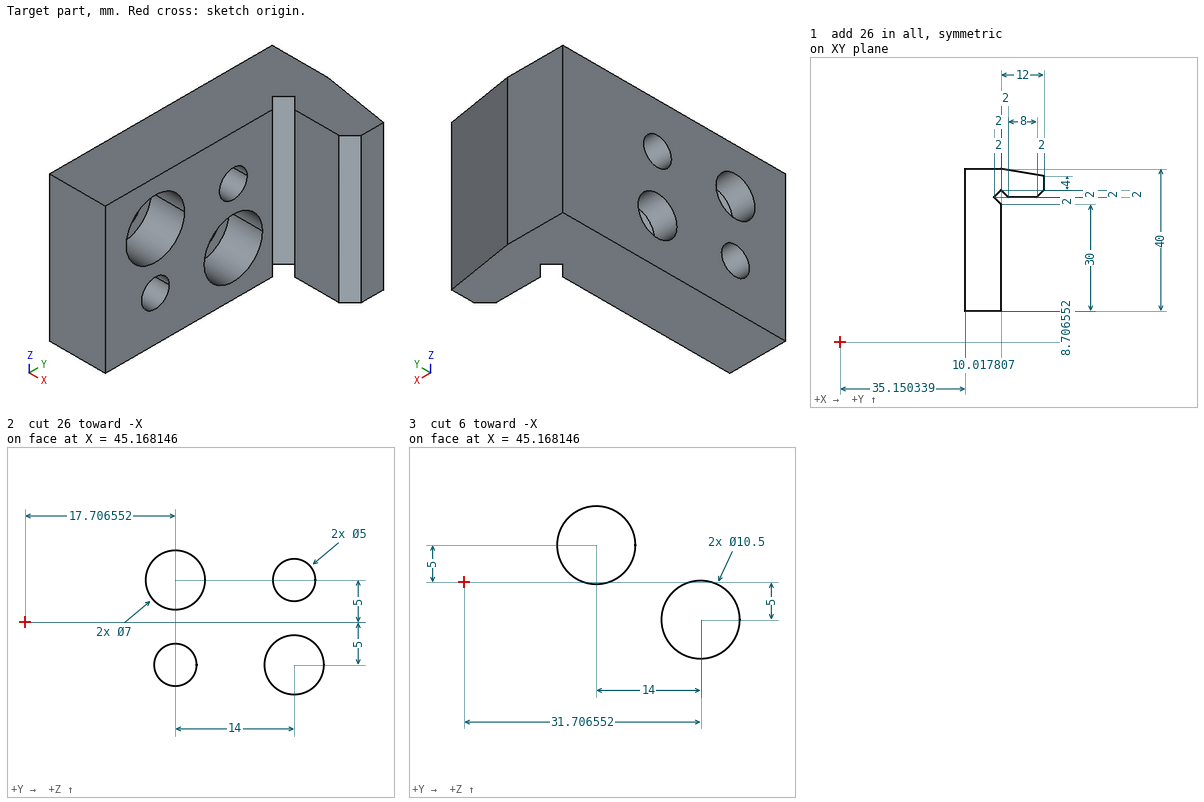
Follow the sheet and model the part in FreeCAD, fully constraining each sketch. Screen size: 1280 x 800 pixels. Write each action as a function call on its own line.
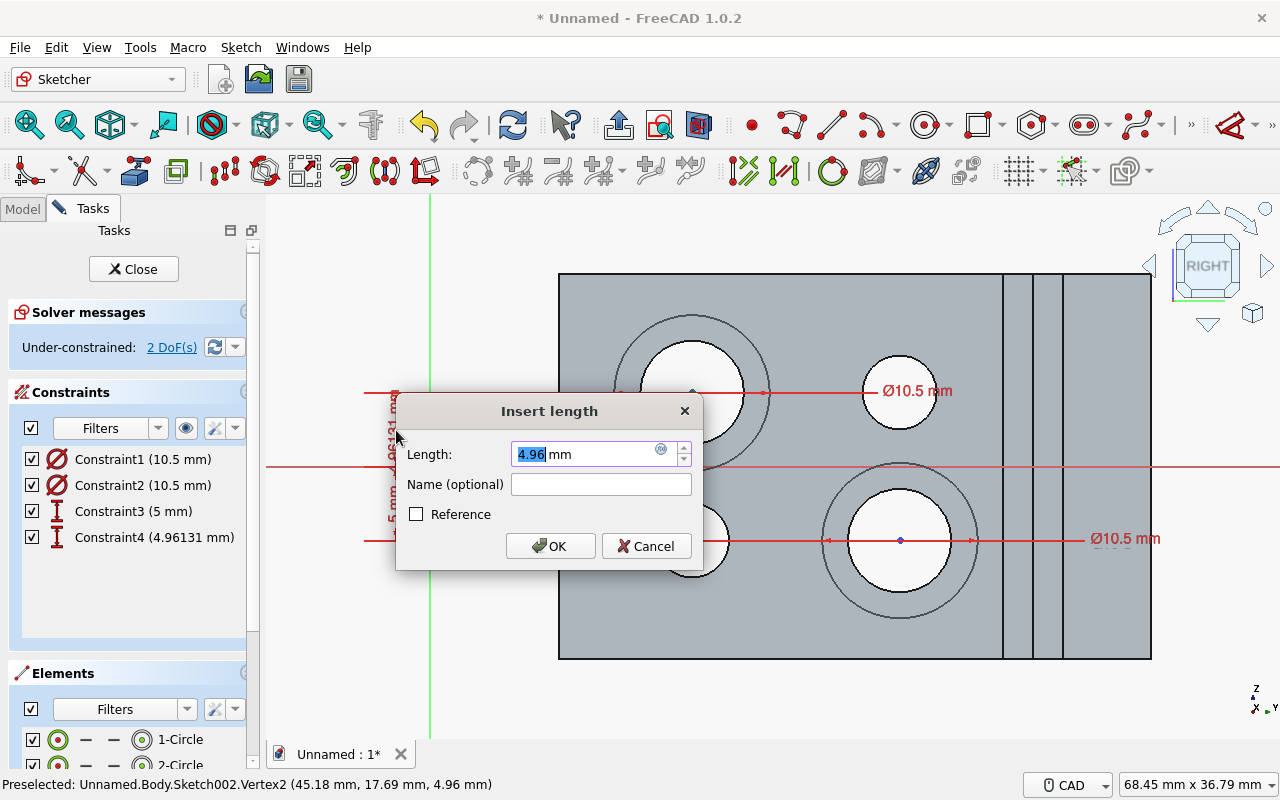
text(5)
key(Return)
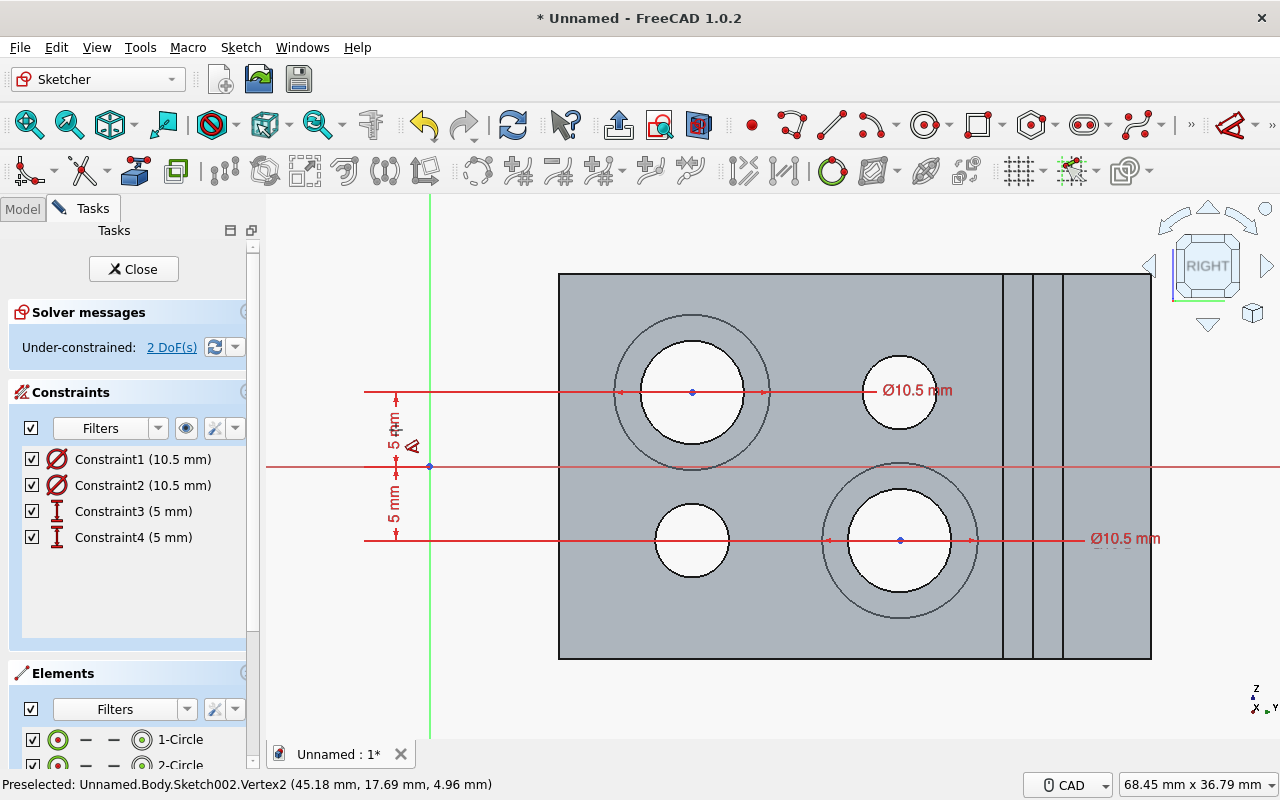
click(900, 541)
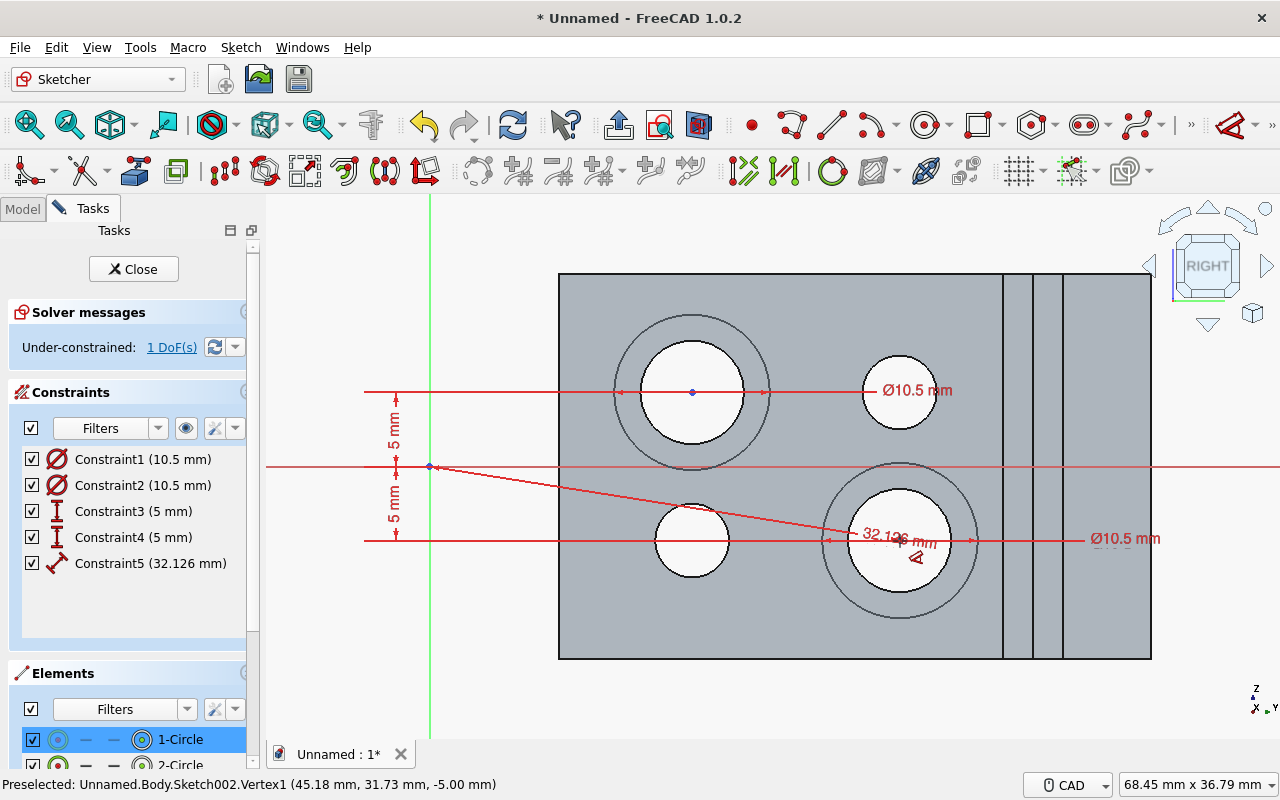
click(692, 392)
click(796, 575)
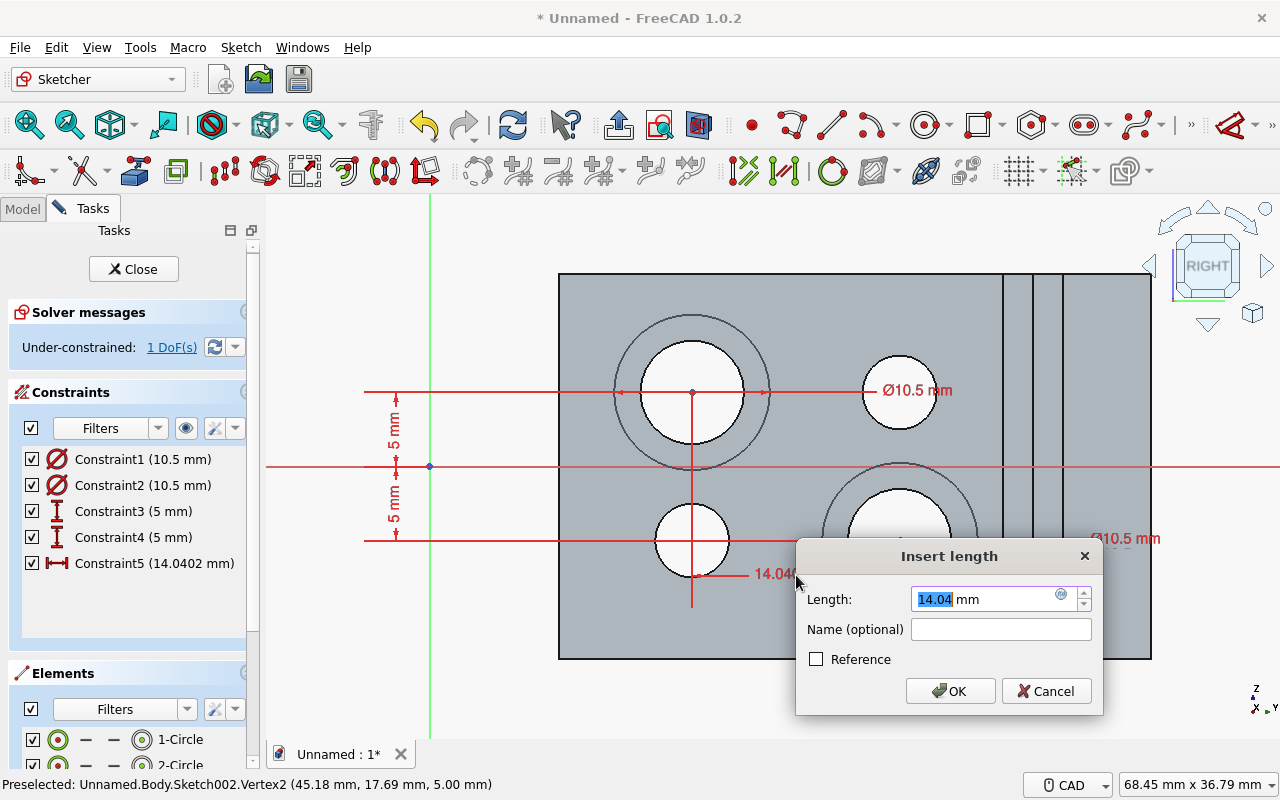
text(14)
key(Return)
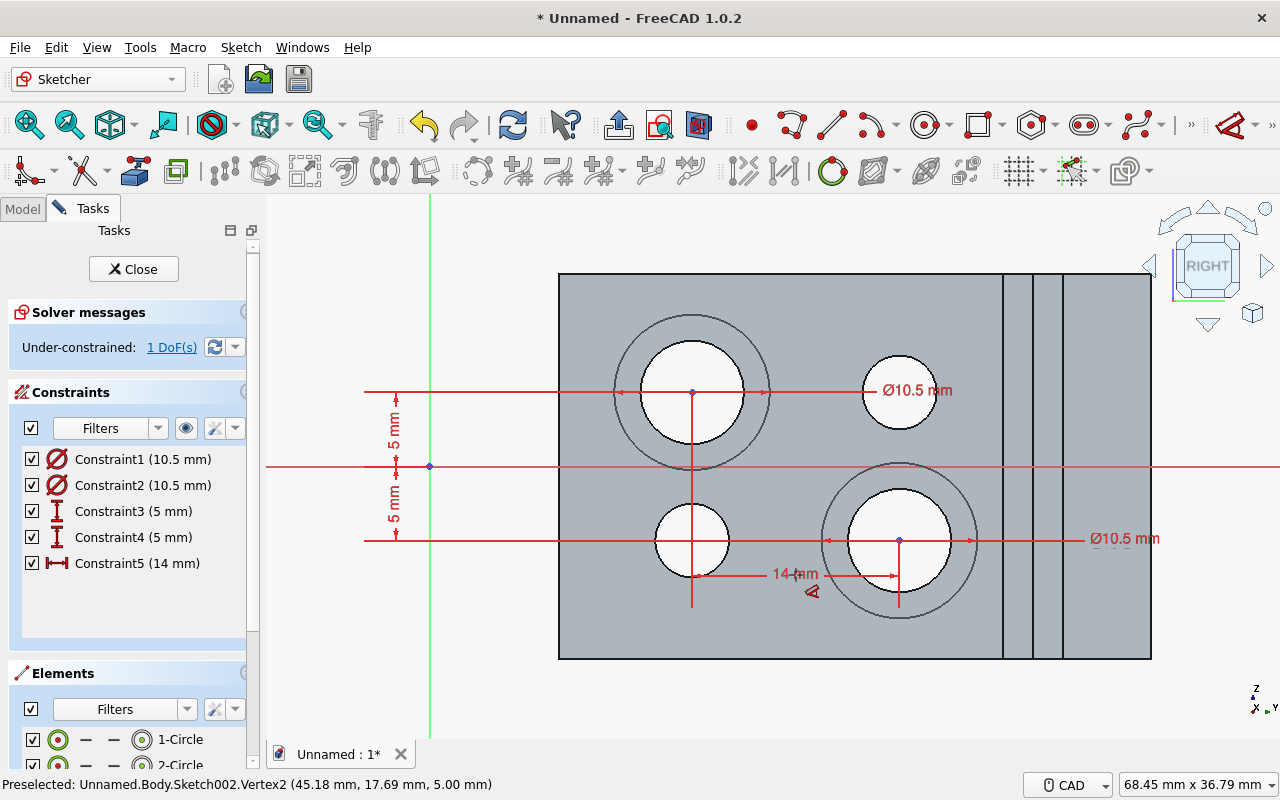
click(899, 541)
click(665, 575)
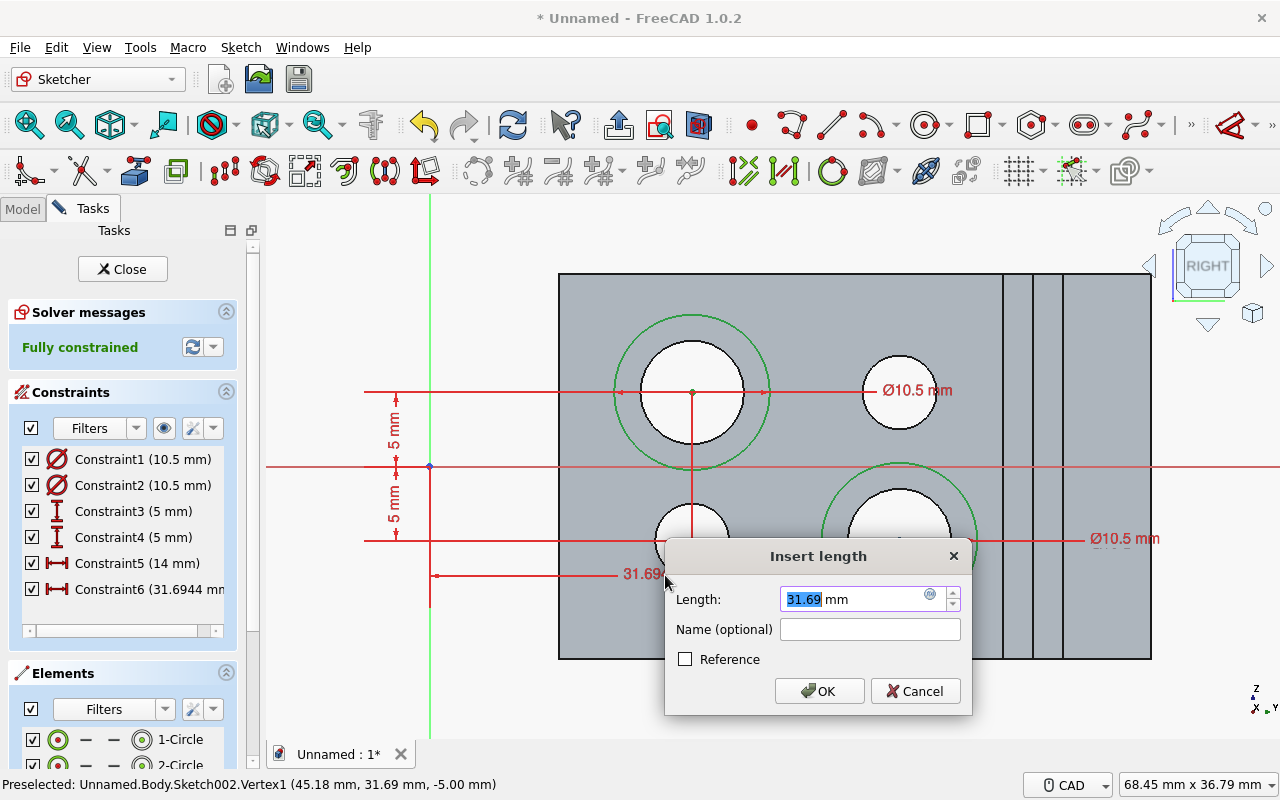
text(31.706552)
key(Return)
key(Escape)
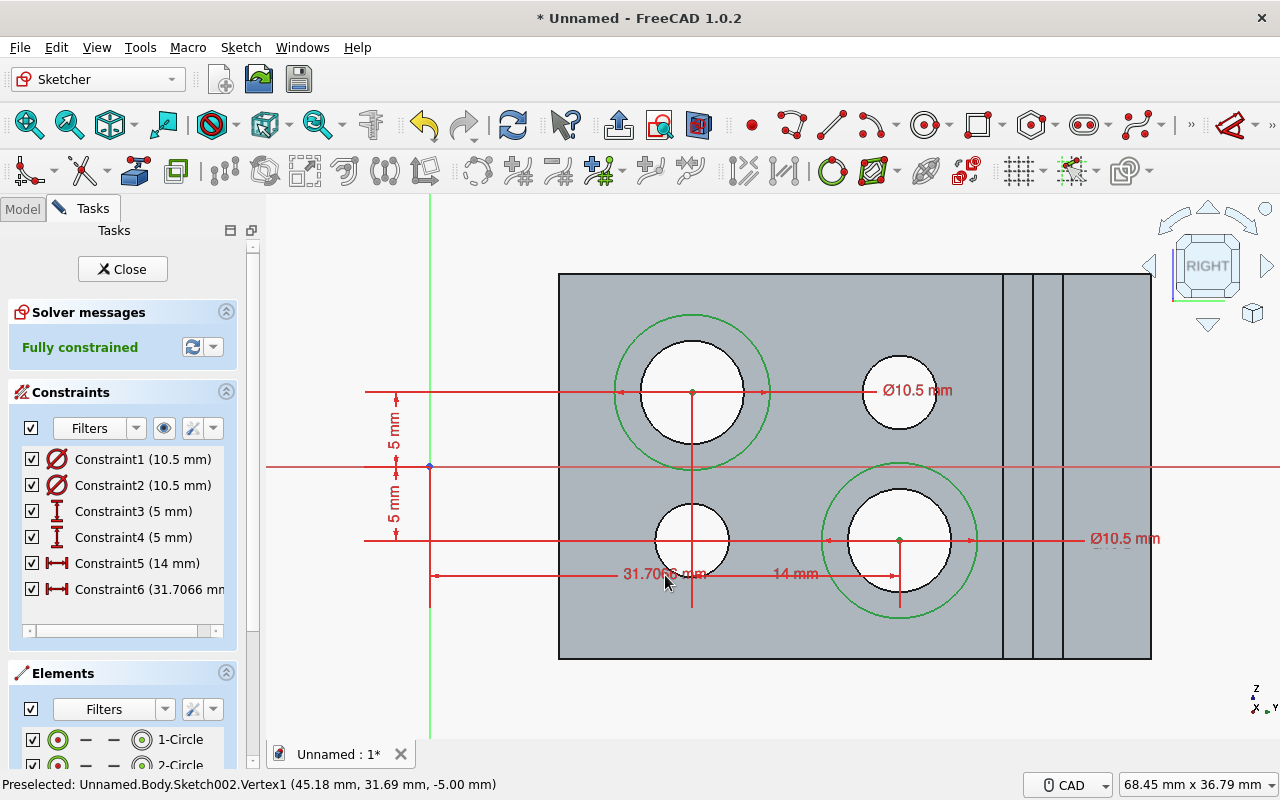
click(123, 269)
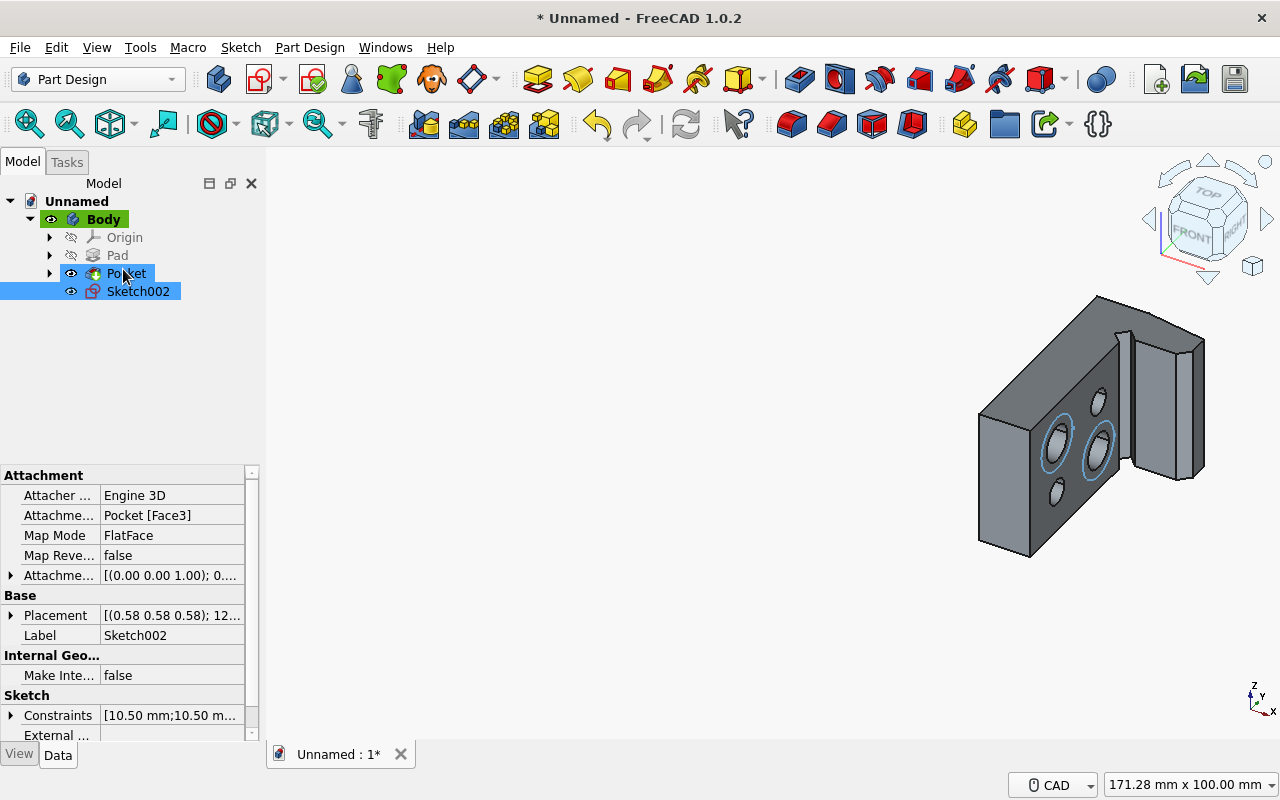
click(800, 80)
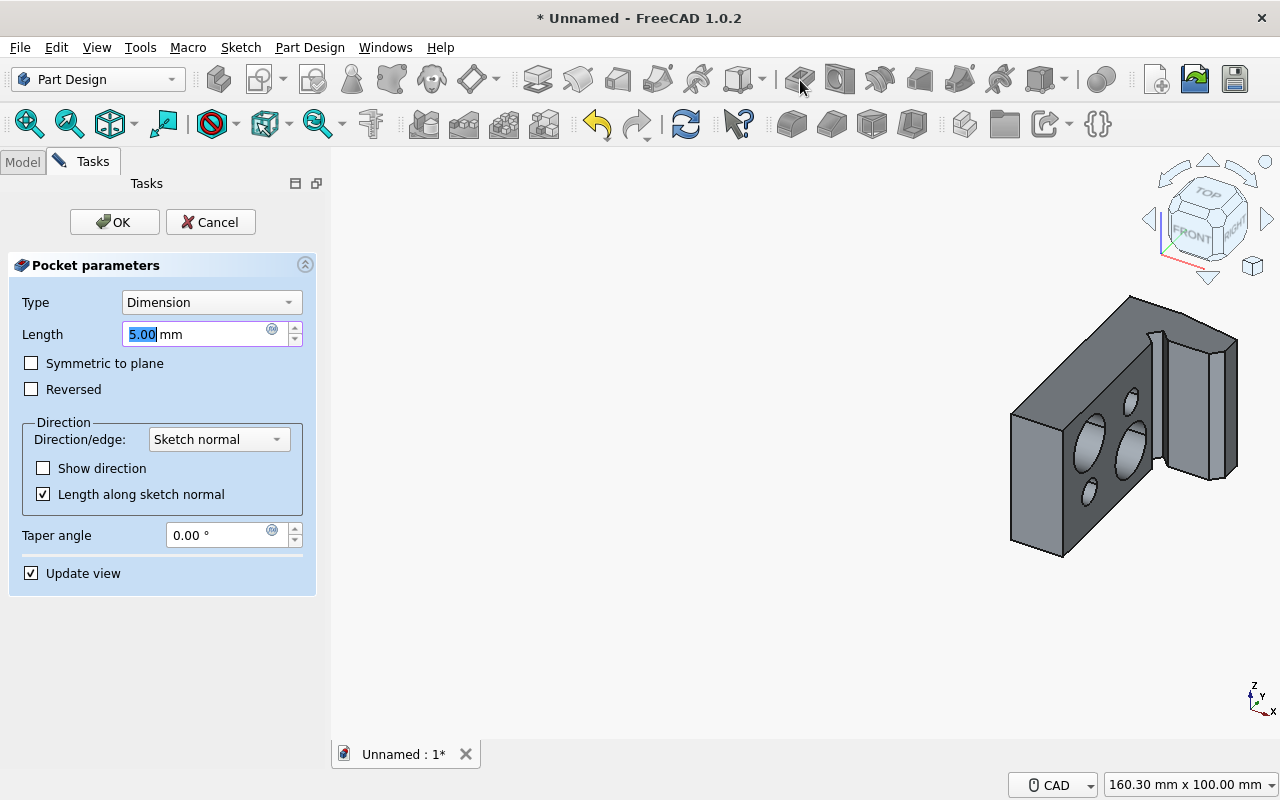
text(6)
key(Tab)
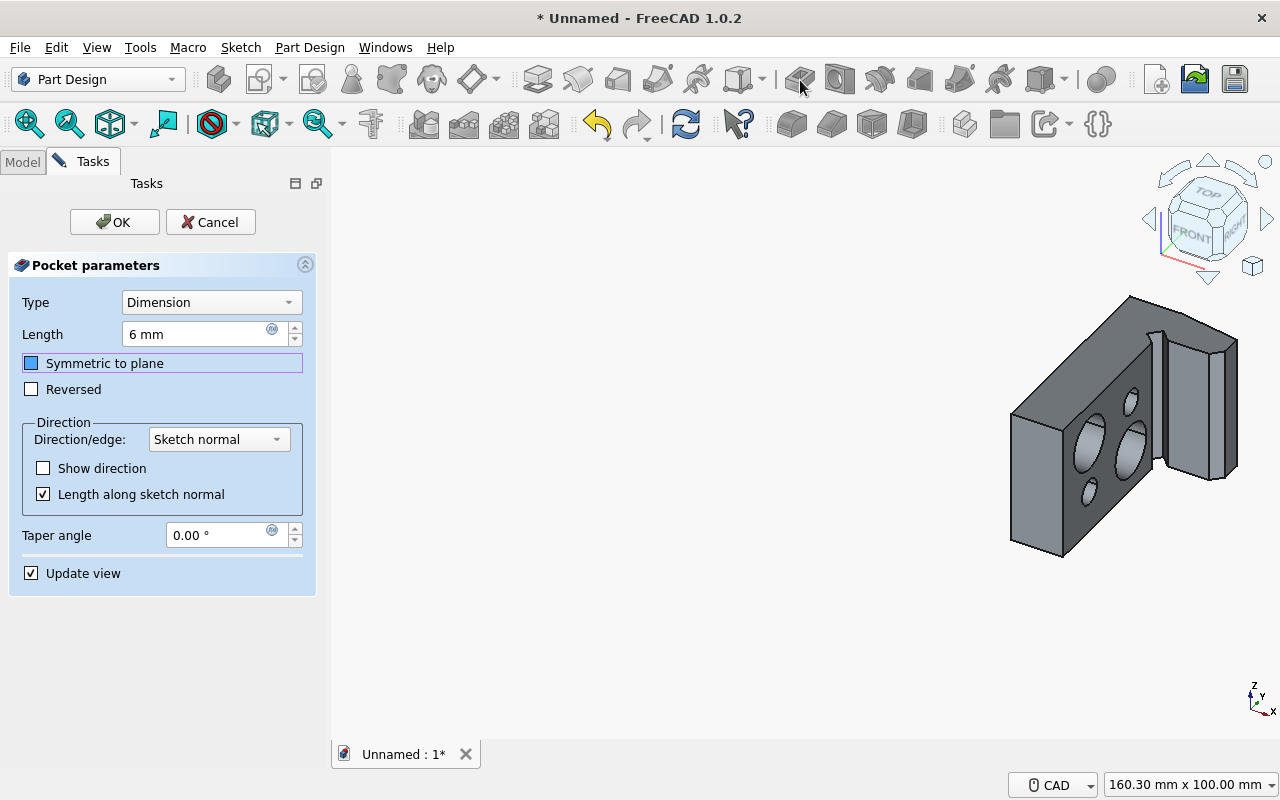
click(115, 222)